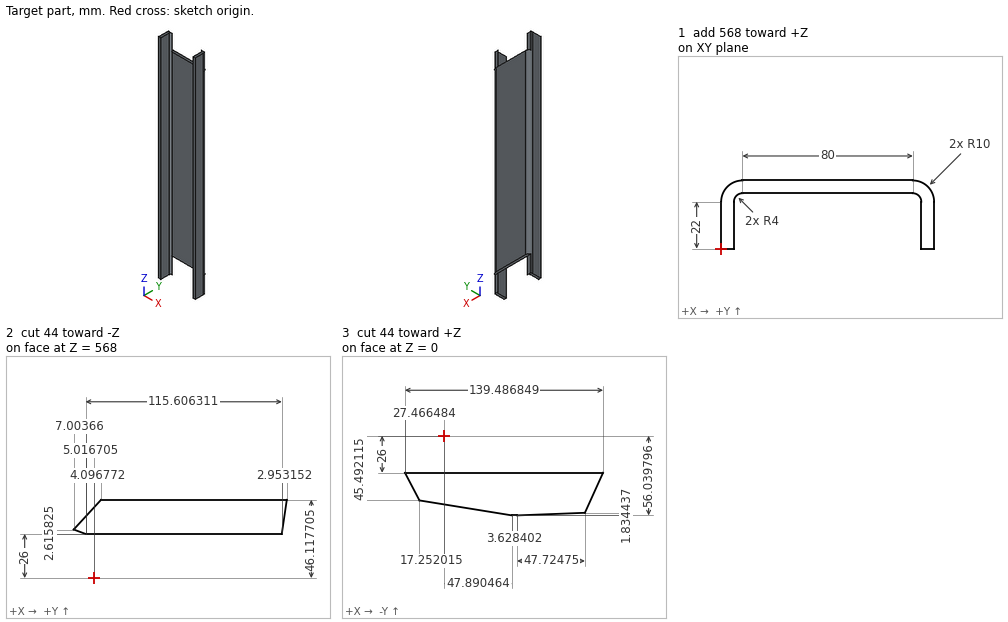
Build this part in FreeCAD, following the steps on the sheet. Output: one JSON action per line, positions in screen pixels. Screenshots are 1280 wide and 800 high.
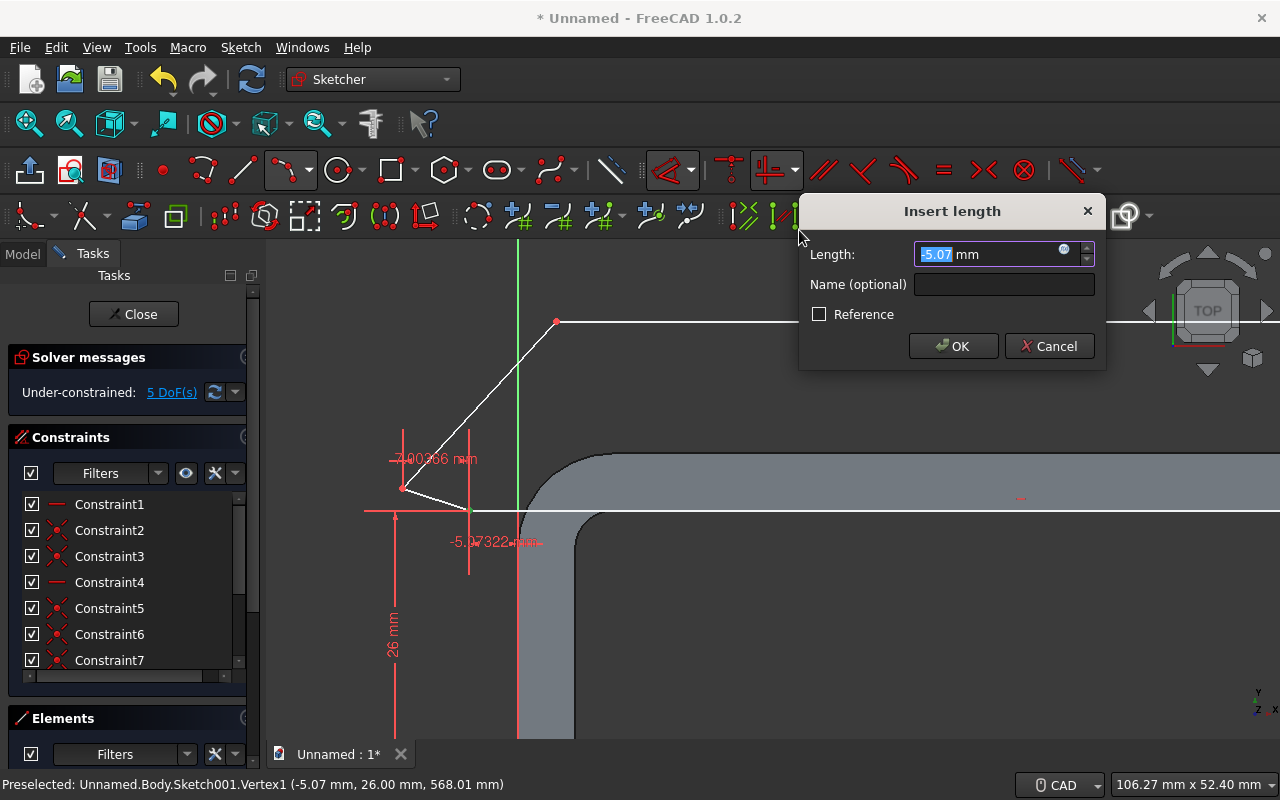
{"action": "type", "text": "-5.016705"}
{"action": "key", "text": "Return"}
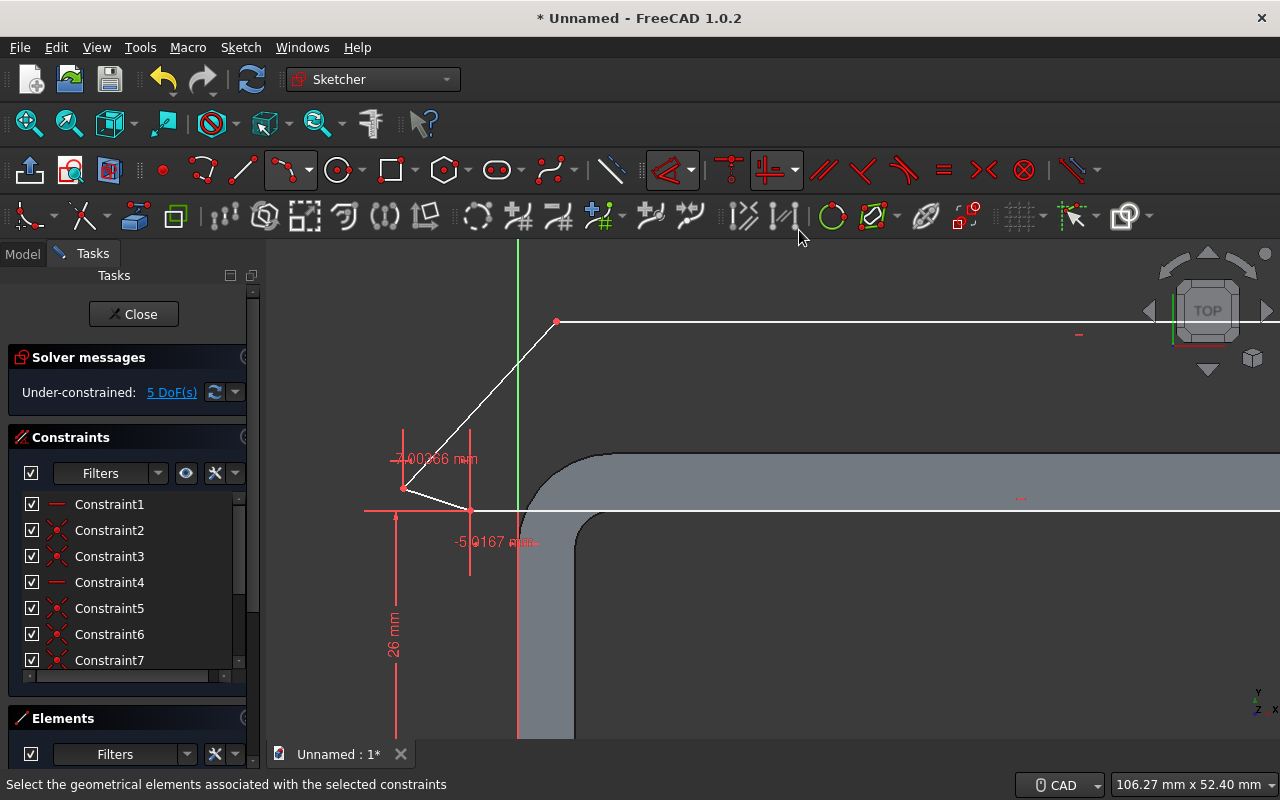
{"action": "left_click", "coordinate": [556, 322]}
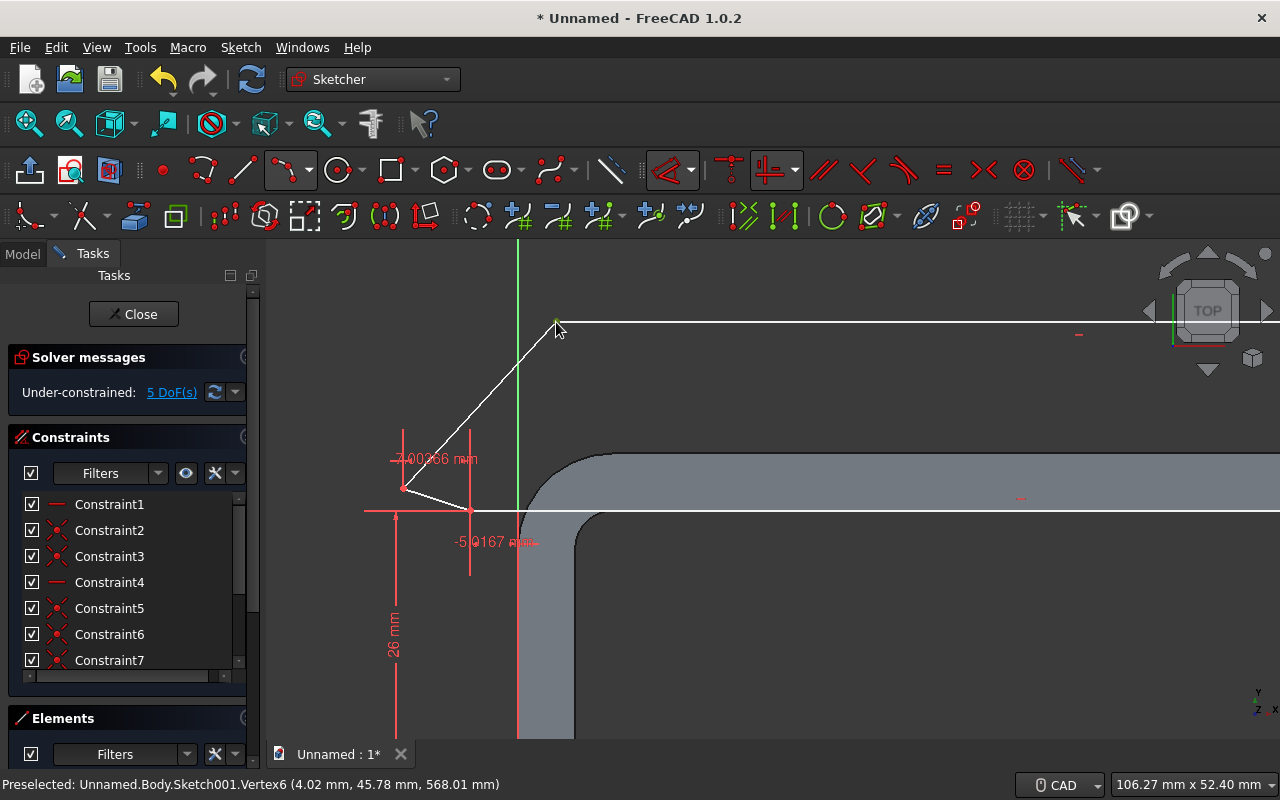
{"action": "left_click", "coordinate": [694, 170]}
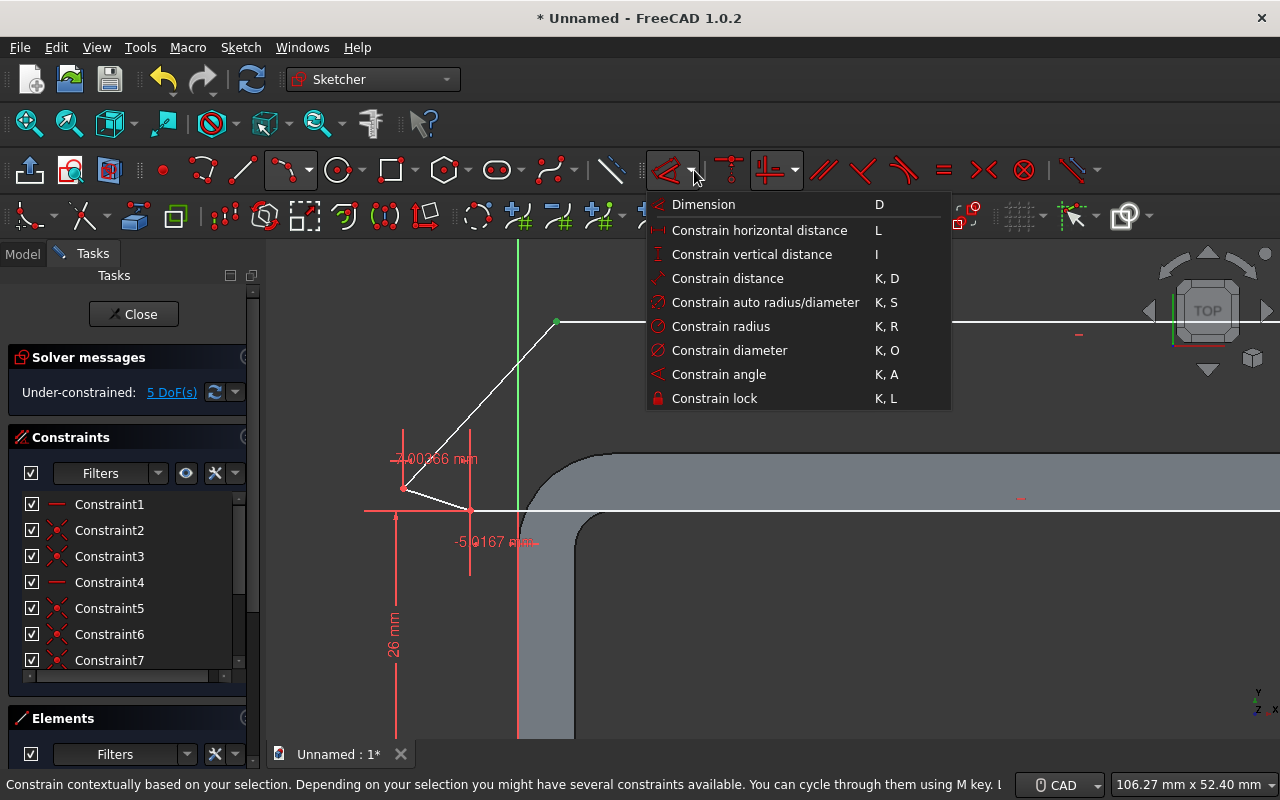
{"action": "left_click", "coordinate": [799, 230]}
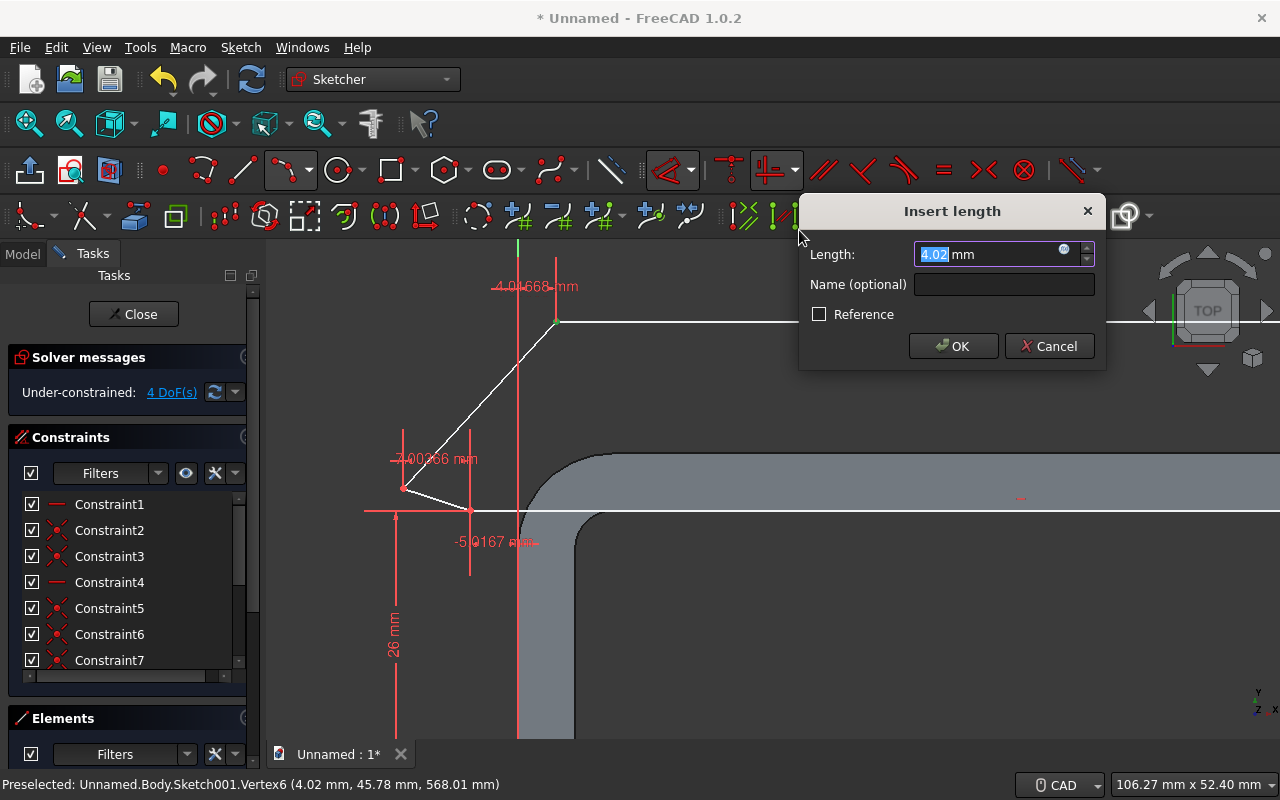
{"action": "type", "text": "4.096772"}
{"action": "key", "text": "Return"}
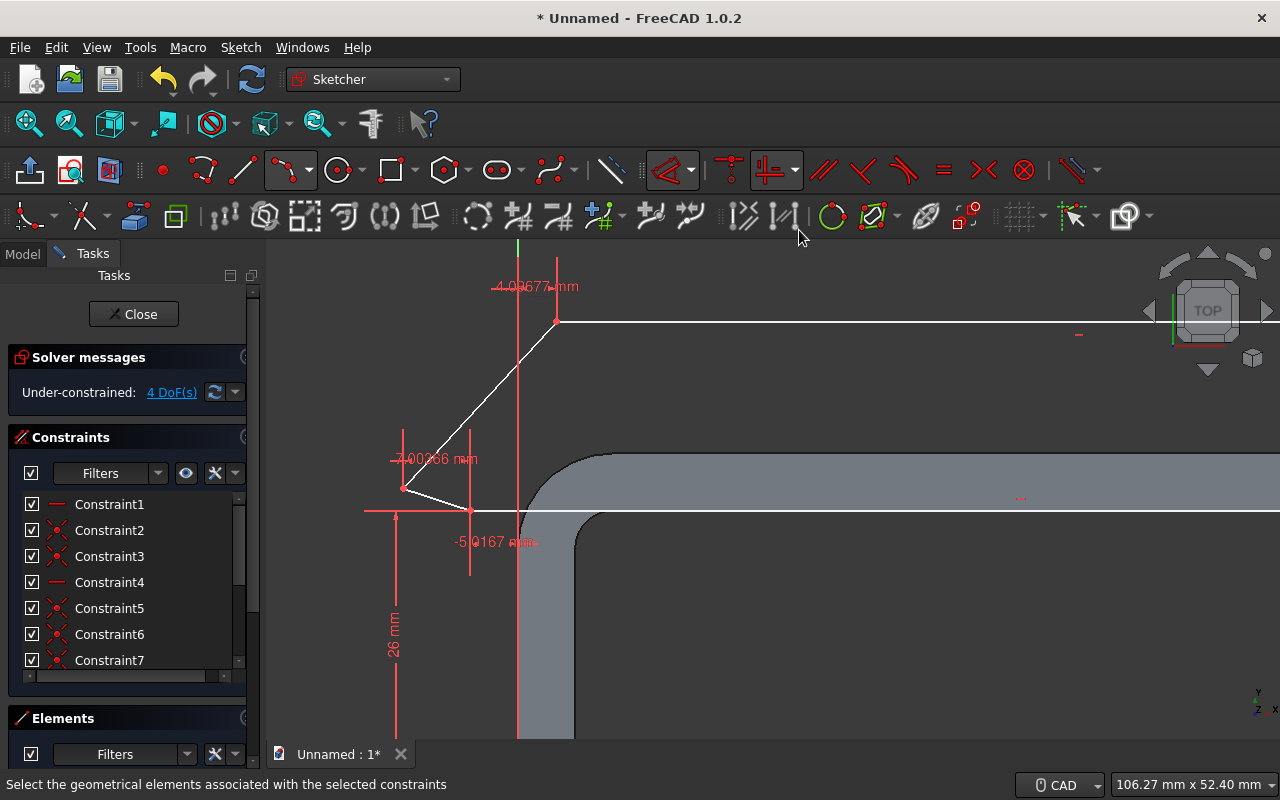
{"action": "scroll", "coordinate": [462, 448], "scroll_direction": "down", "scroll_amount": 4}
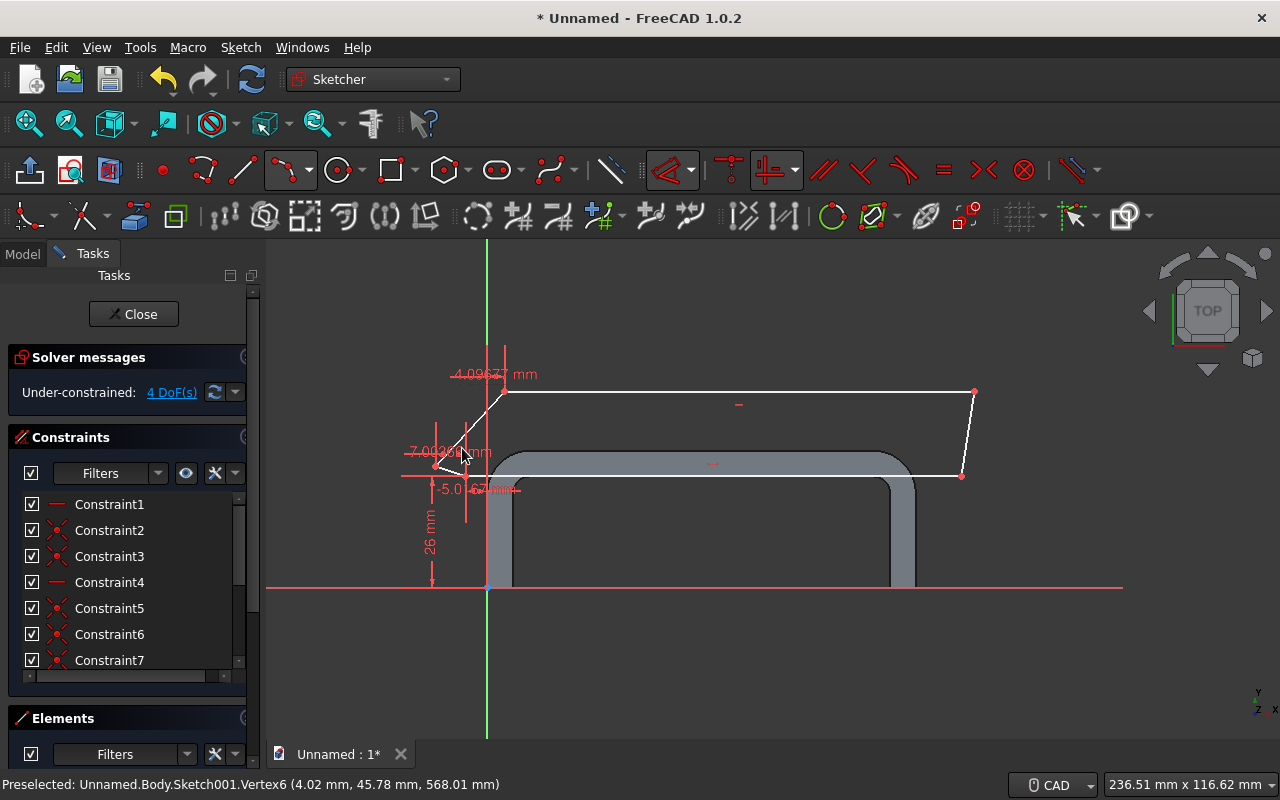
{"action": "scroll", "coordinate": [965, 451], "scroll_direction": "up", "scroll_amount": 6}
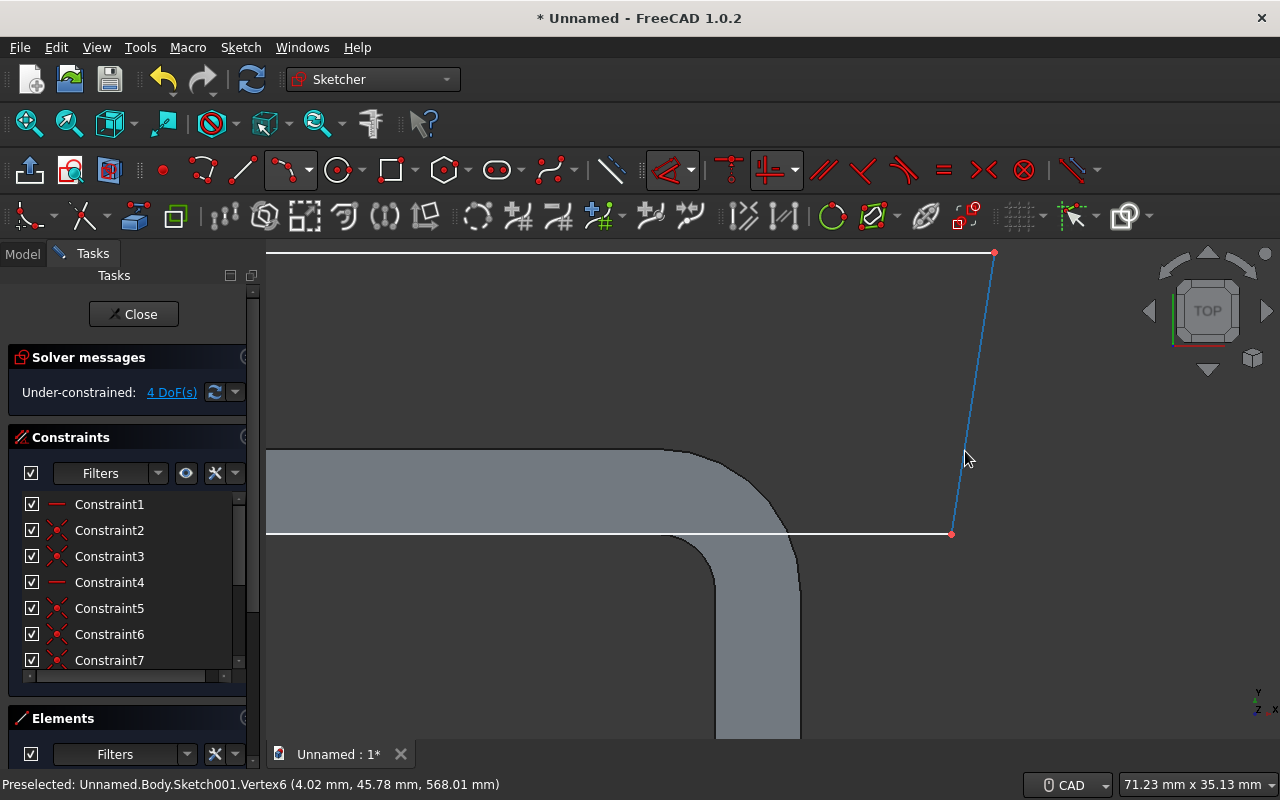
{"action": "left_click", "coordinate": [964, 450]}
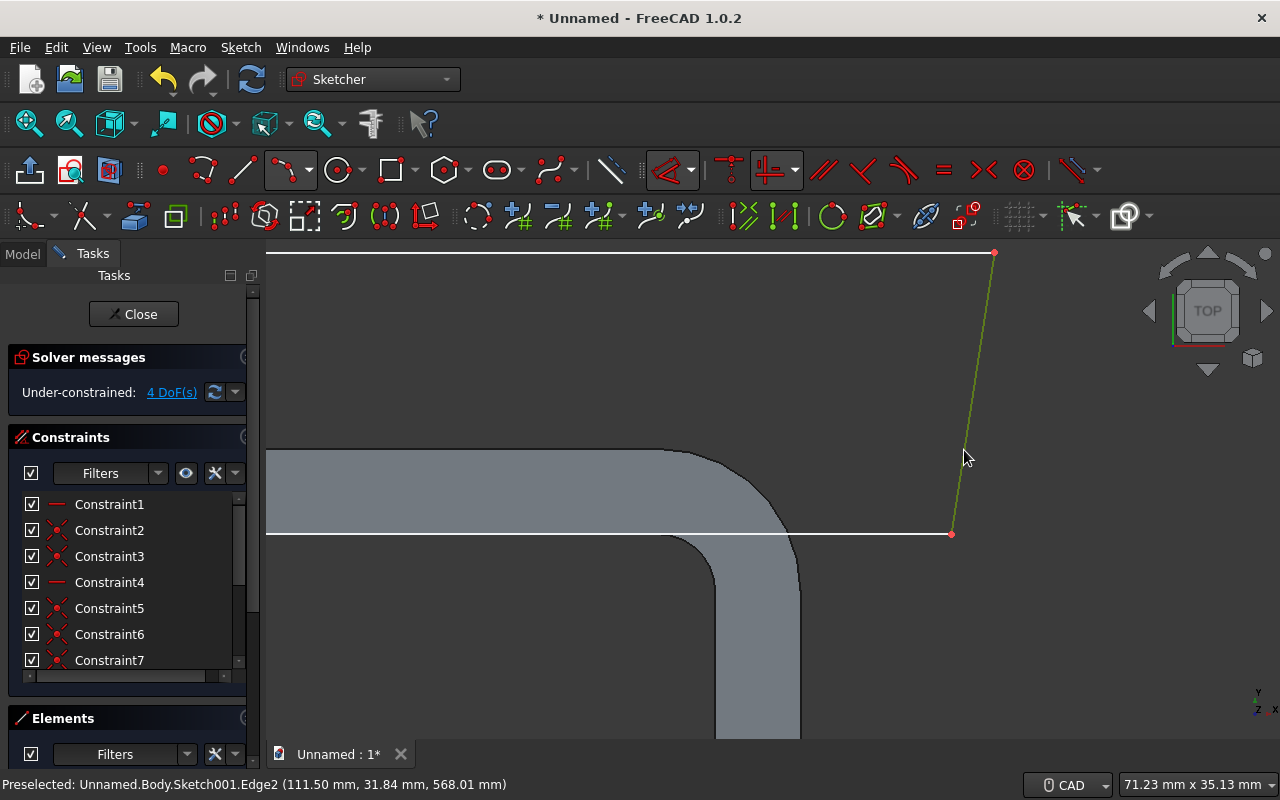
{"action": "left_click", "coordinate": [694, 170]}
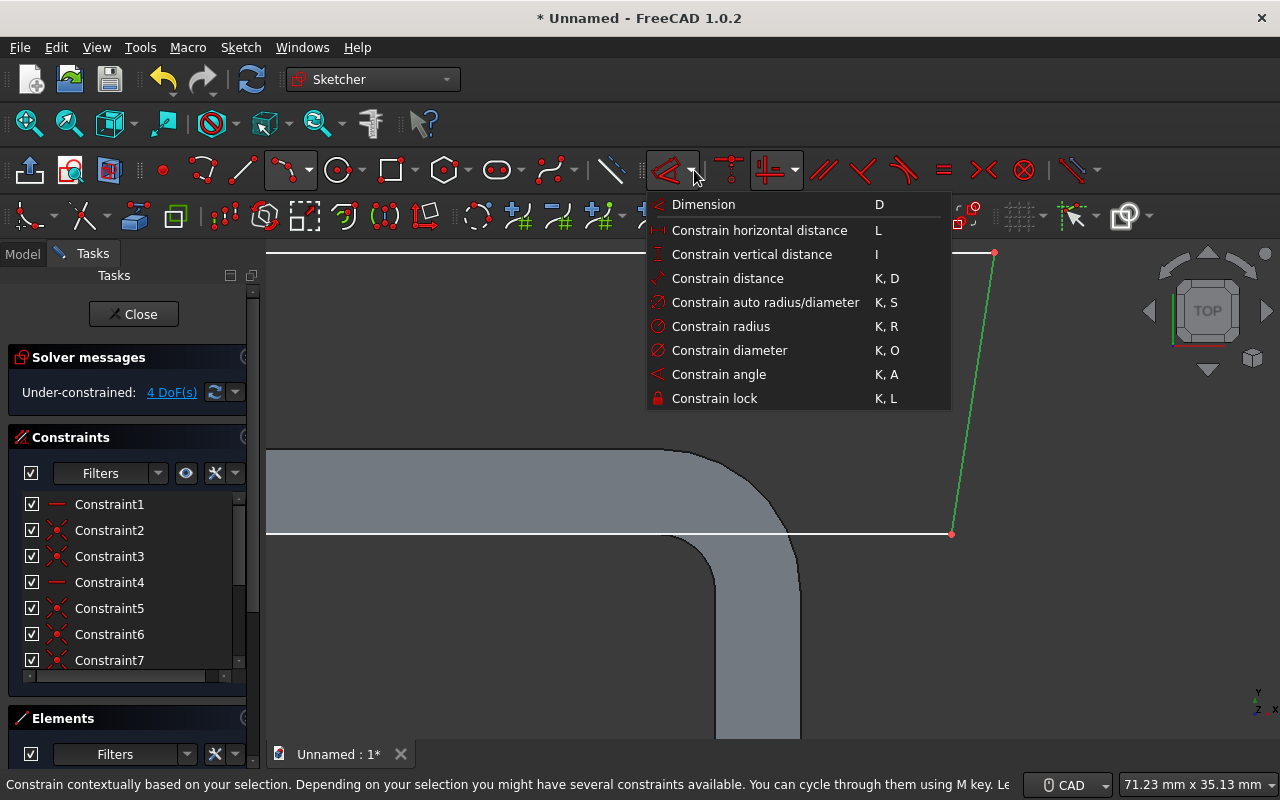
{"action": "left_click", "coordinate": [799, 230]}